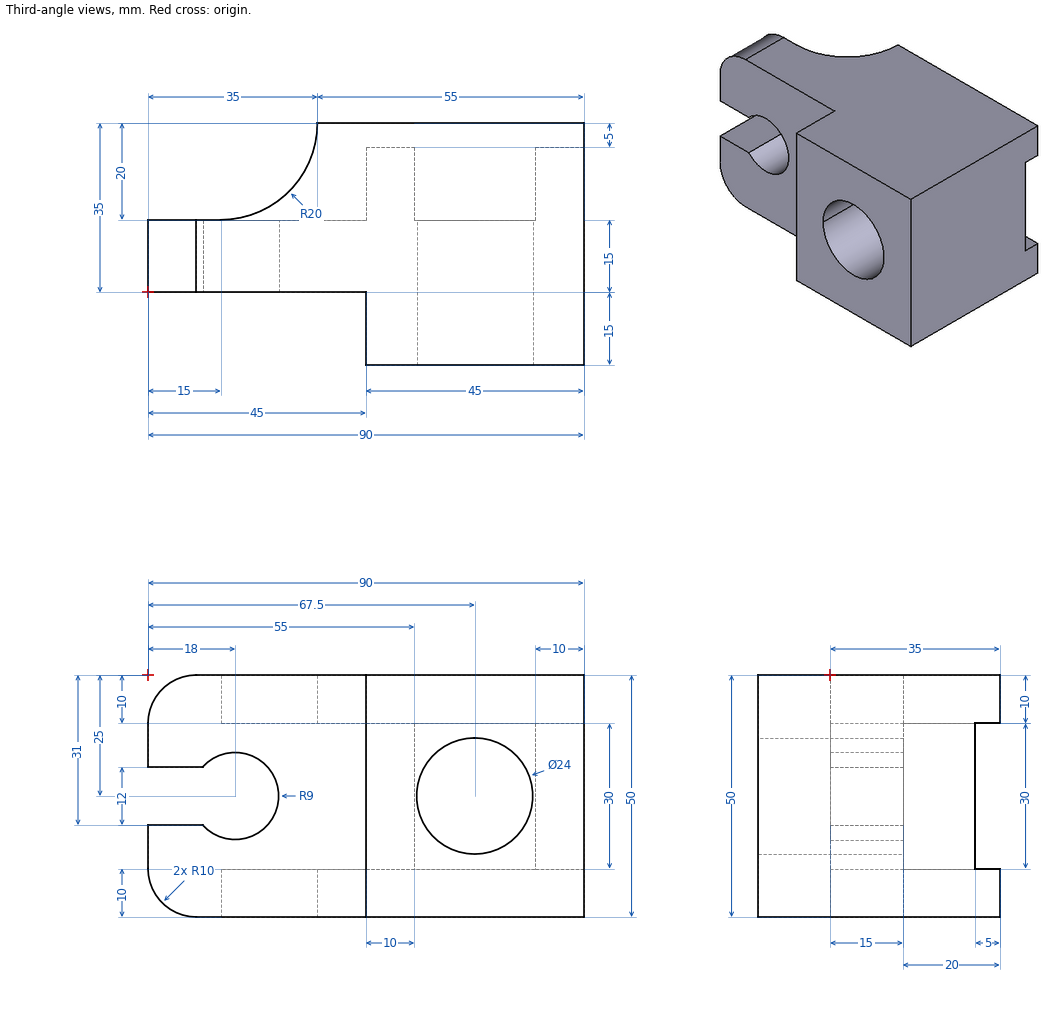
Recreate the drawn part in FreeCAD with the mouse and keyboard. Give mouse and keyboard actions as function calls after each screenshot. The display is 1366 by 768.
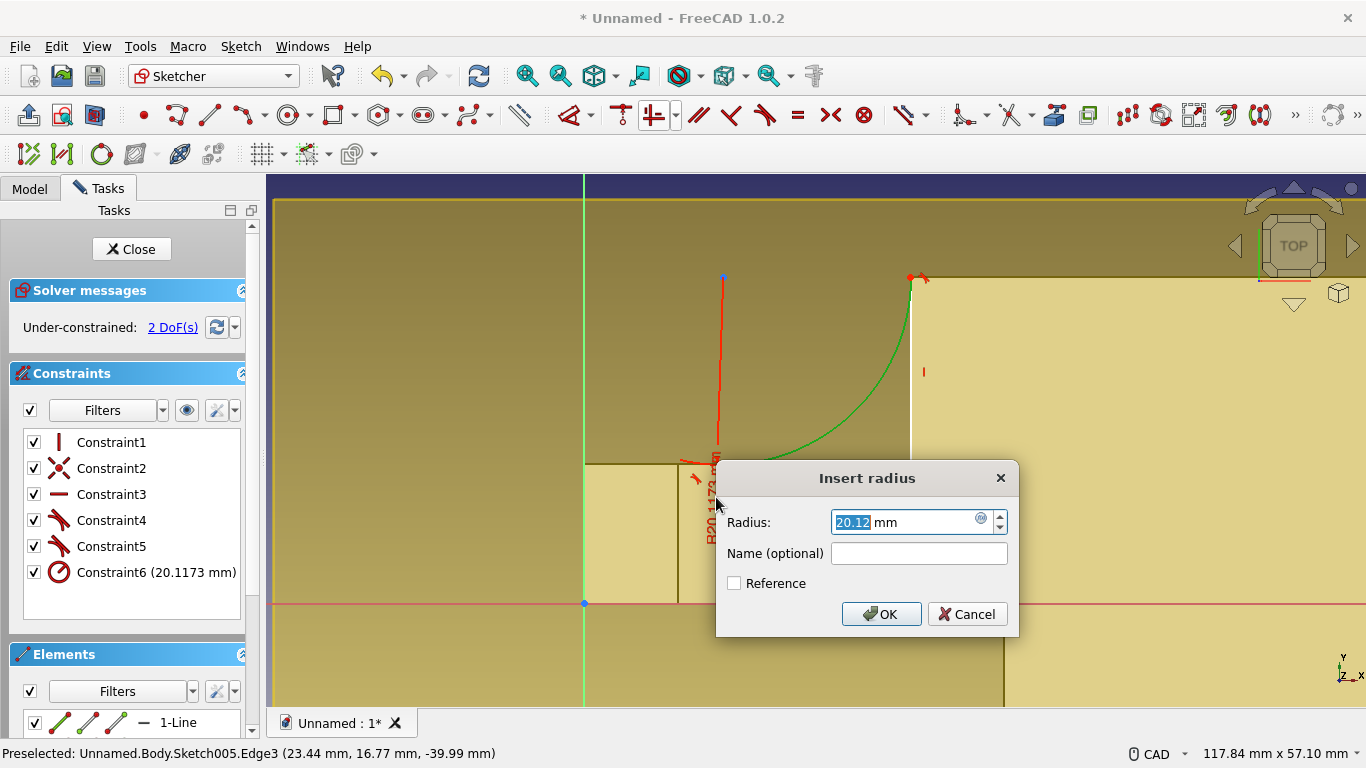
text(20)
key(Return)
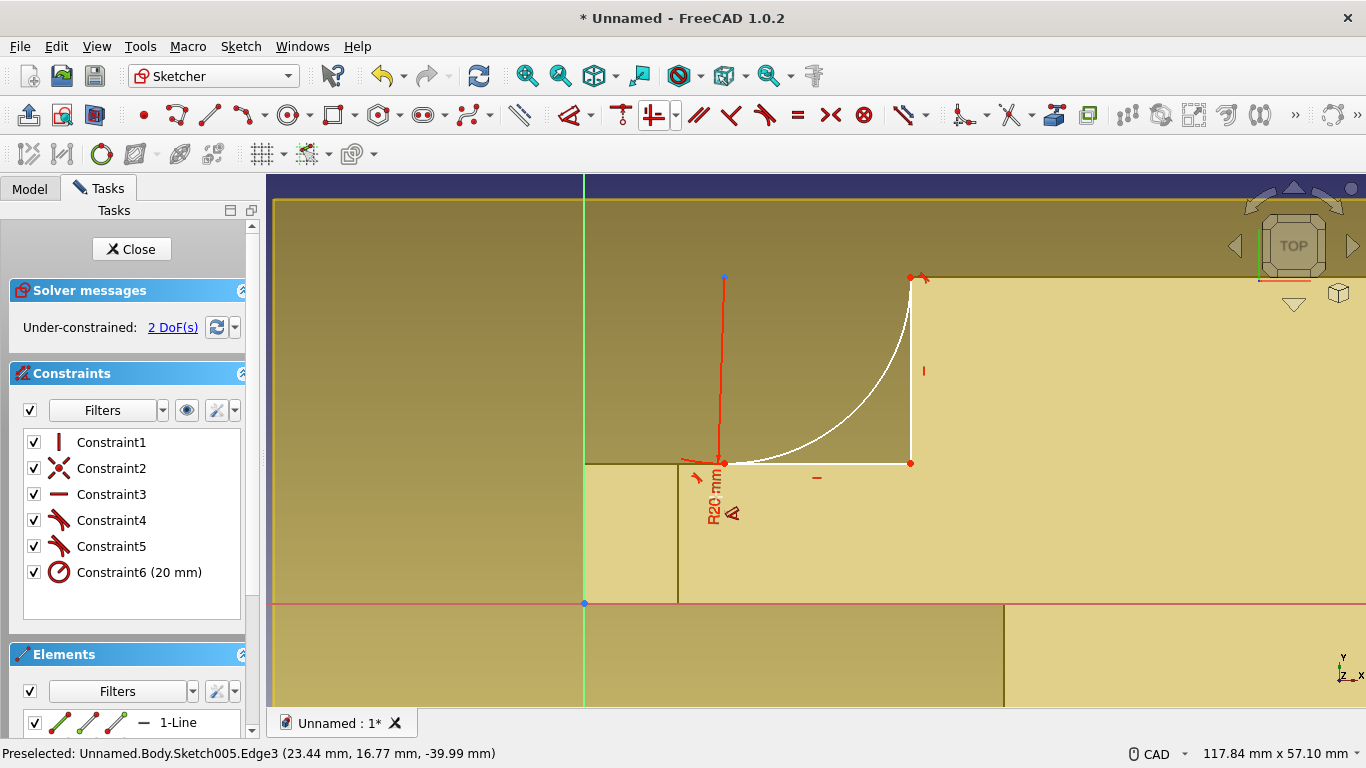
click(911, 277)
click(748, 638)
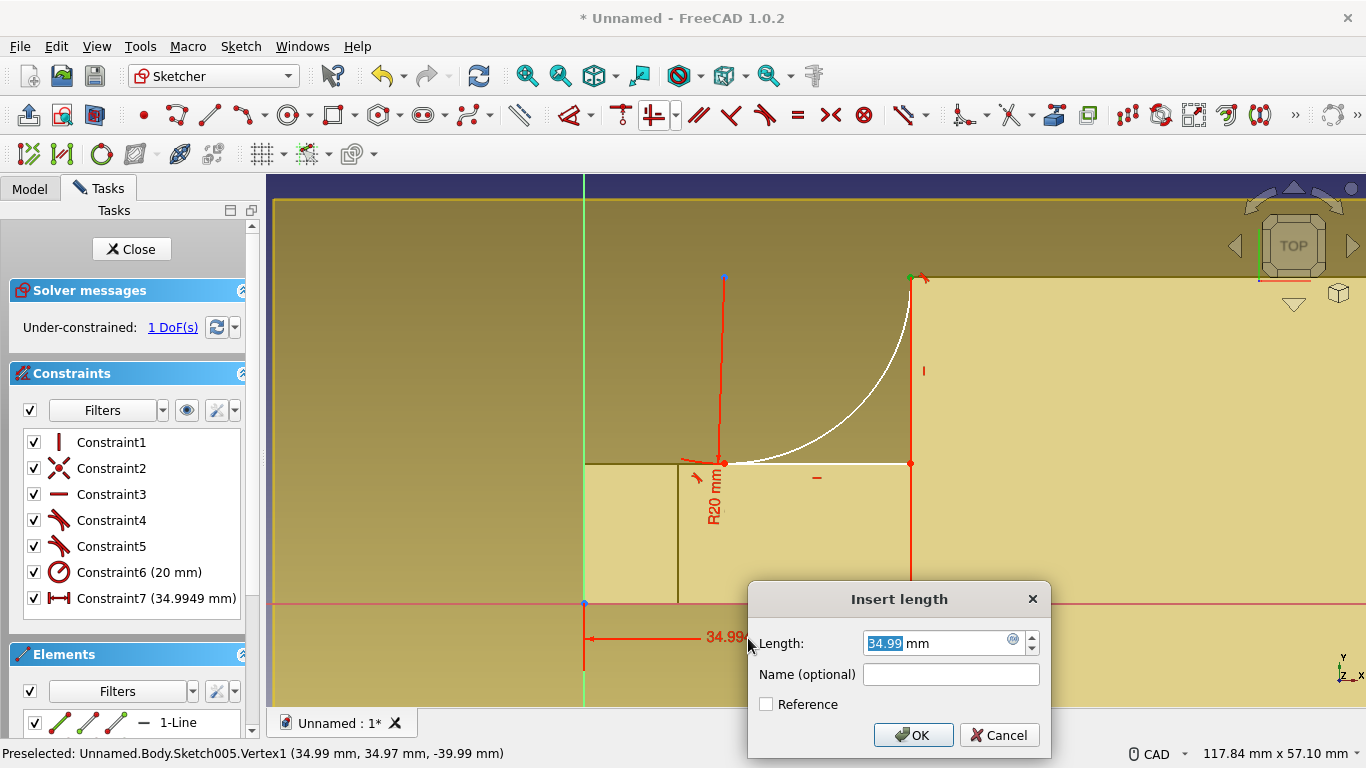
text(35)
key(Return)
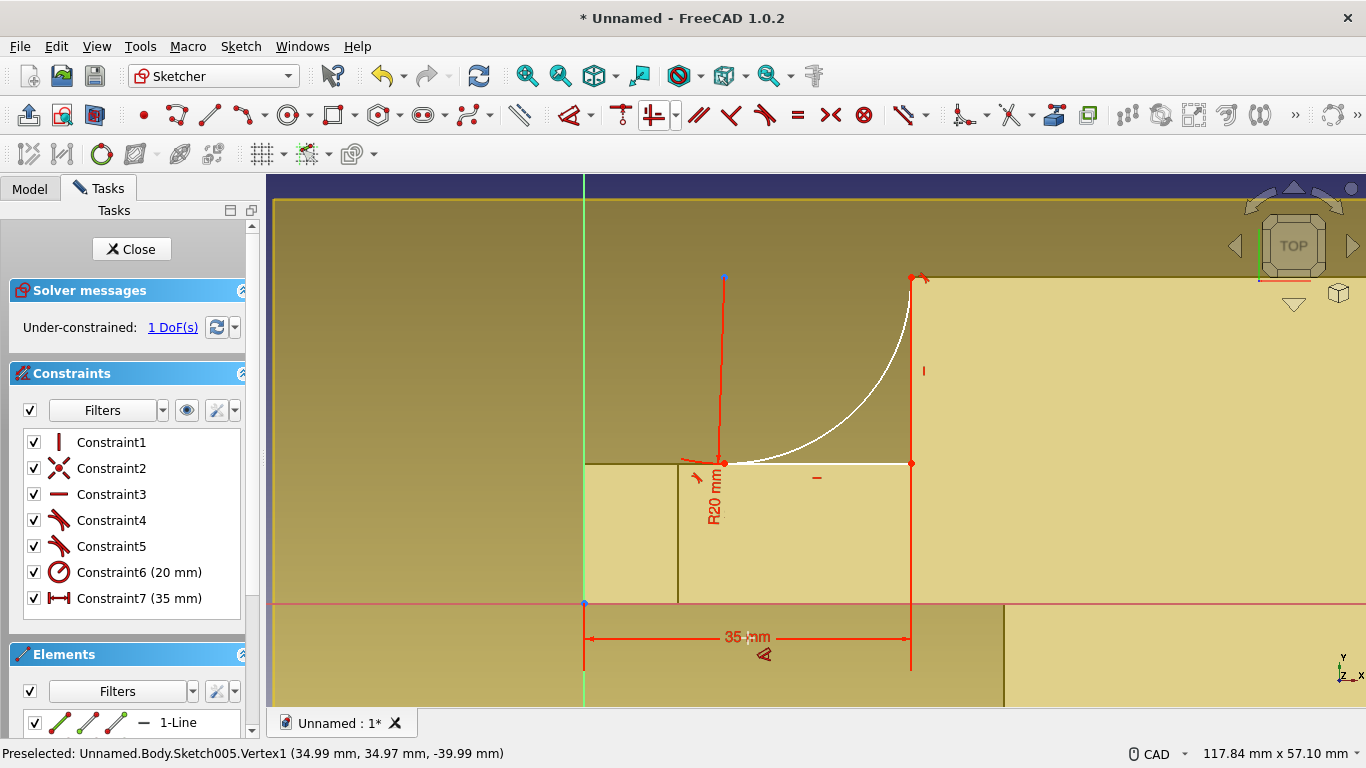
click(911, 277)
click(945, 440)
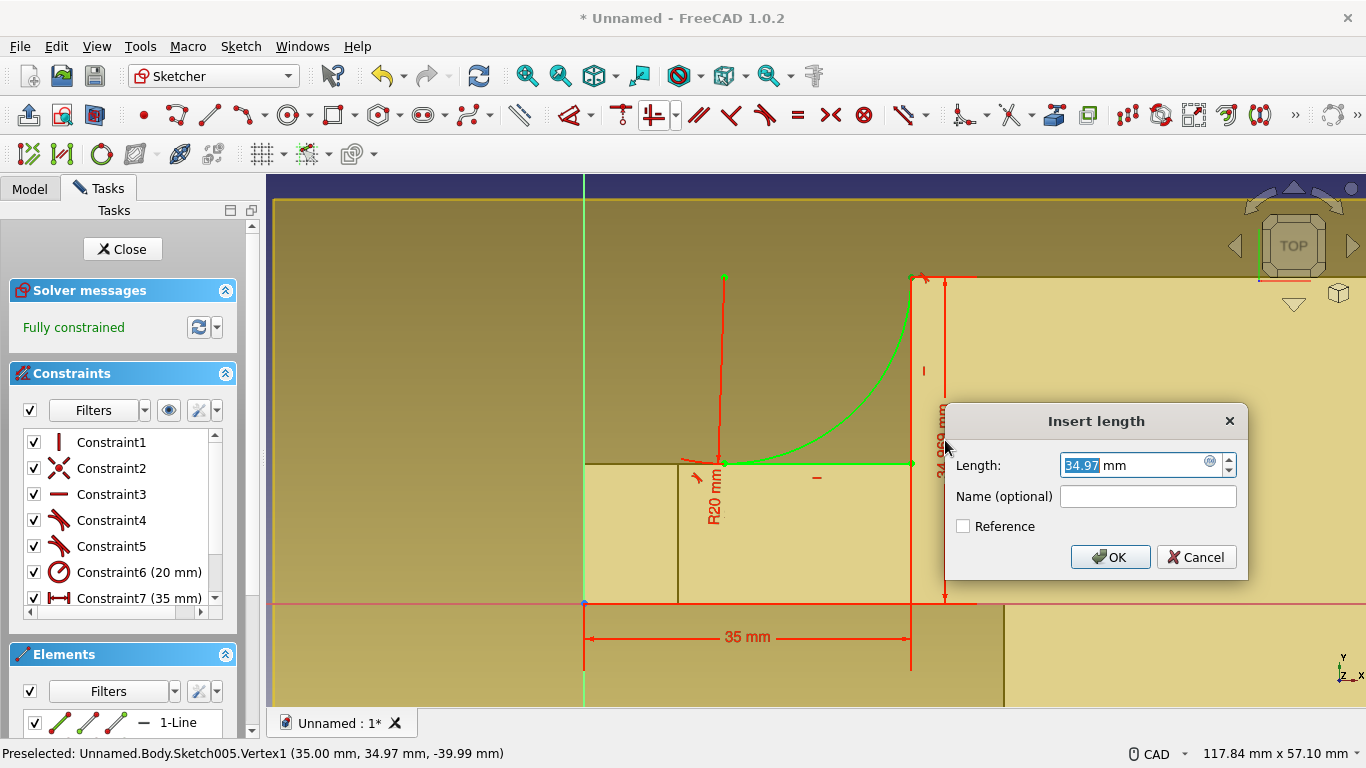
text(35)
key(Return)
key(Escape)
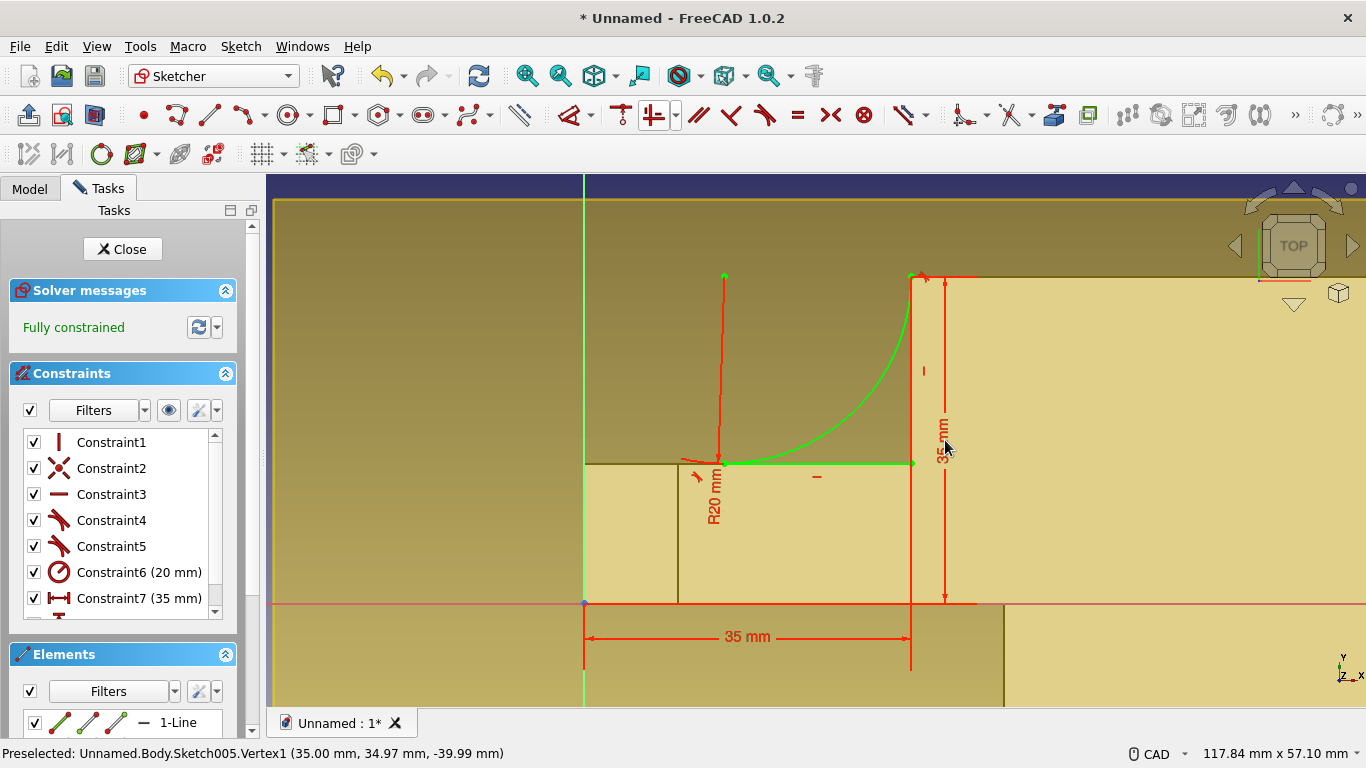
click(123, 249)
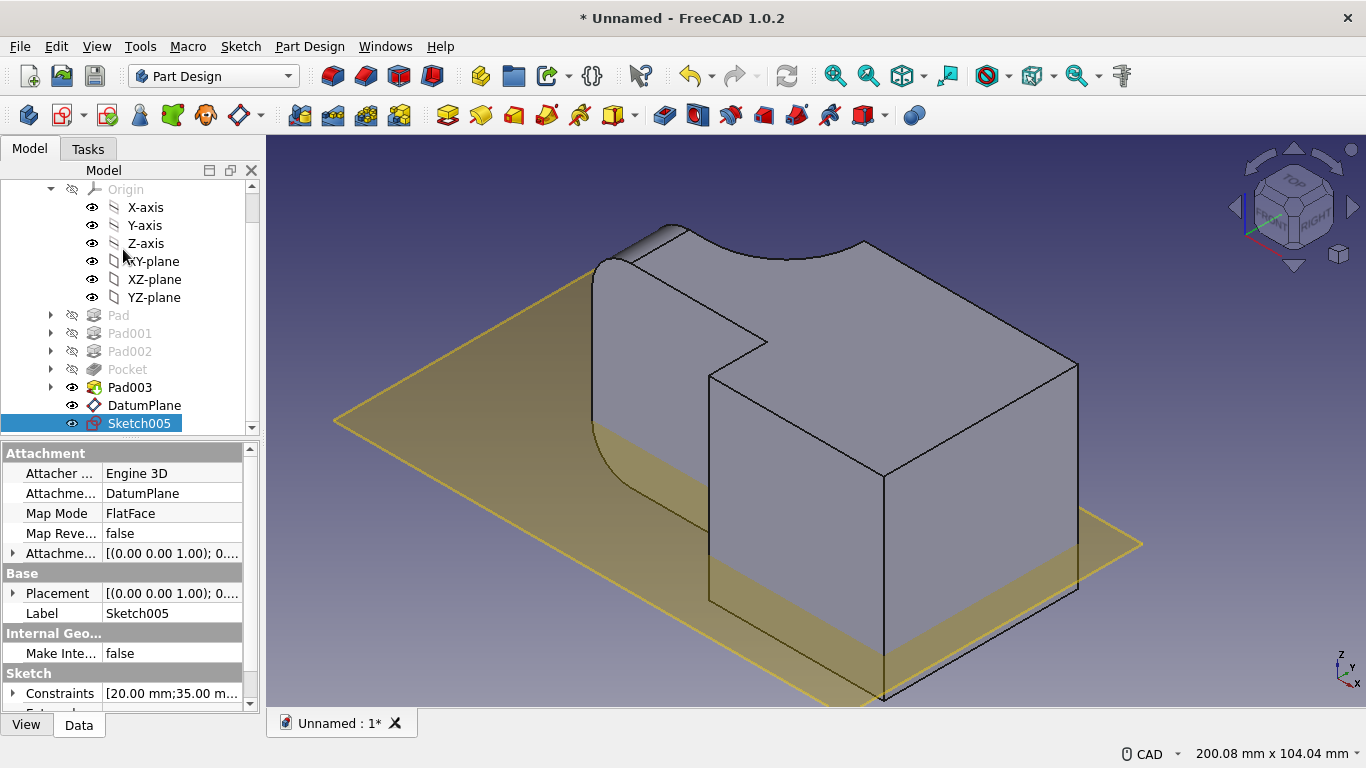
click(448, 116)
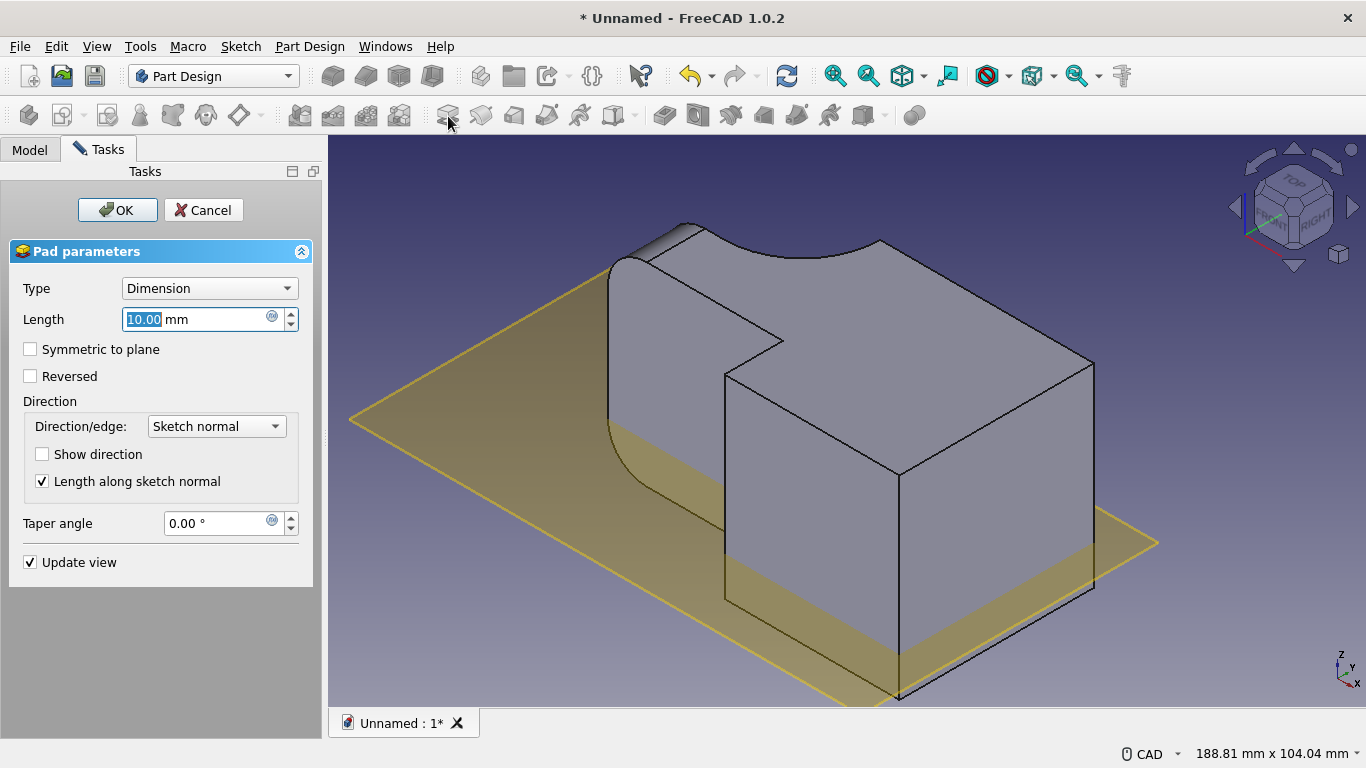
text(10)
key(Tab)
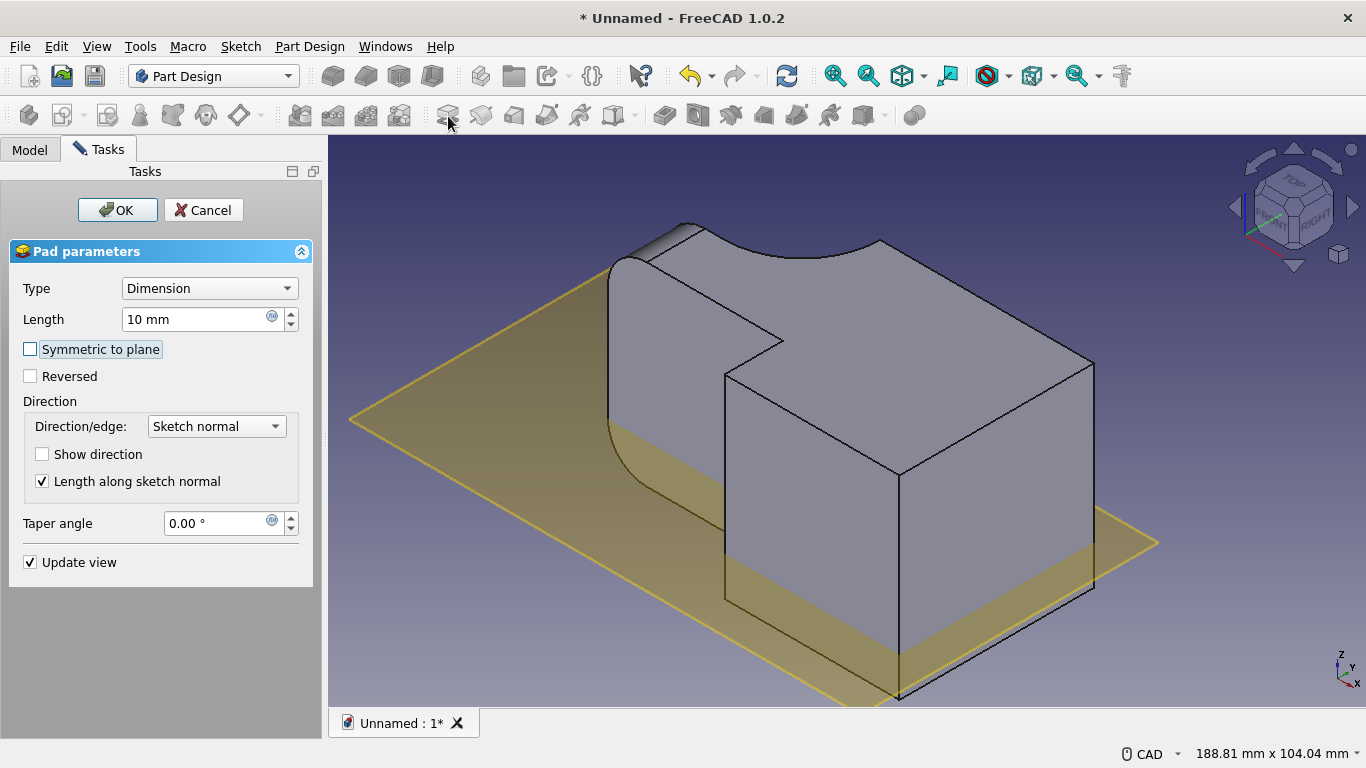
click(31, 376)